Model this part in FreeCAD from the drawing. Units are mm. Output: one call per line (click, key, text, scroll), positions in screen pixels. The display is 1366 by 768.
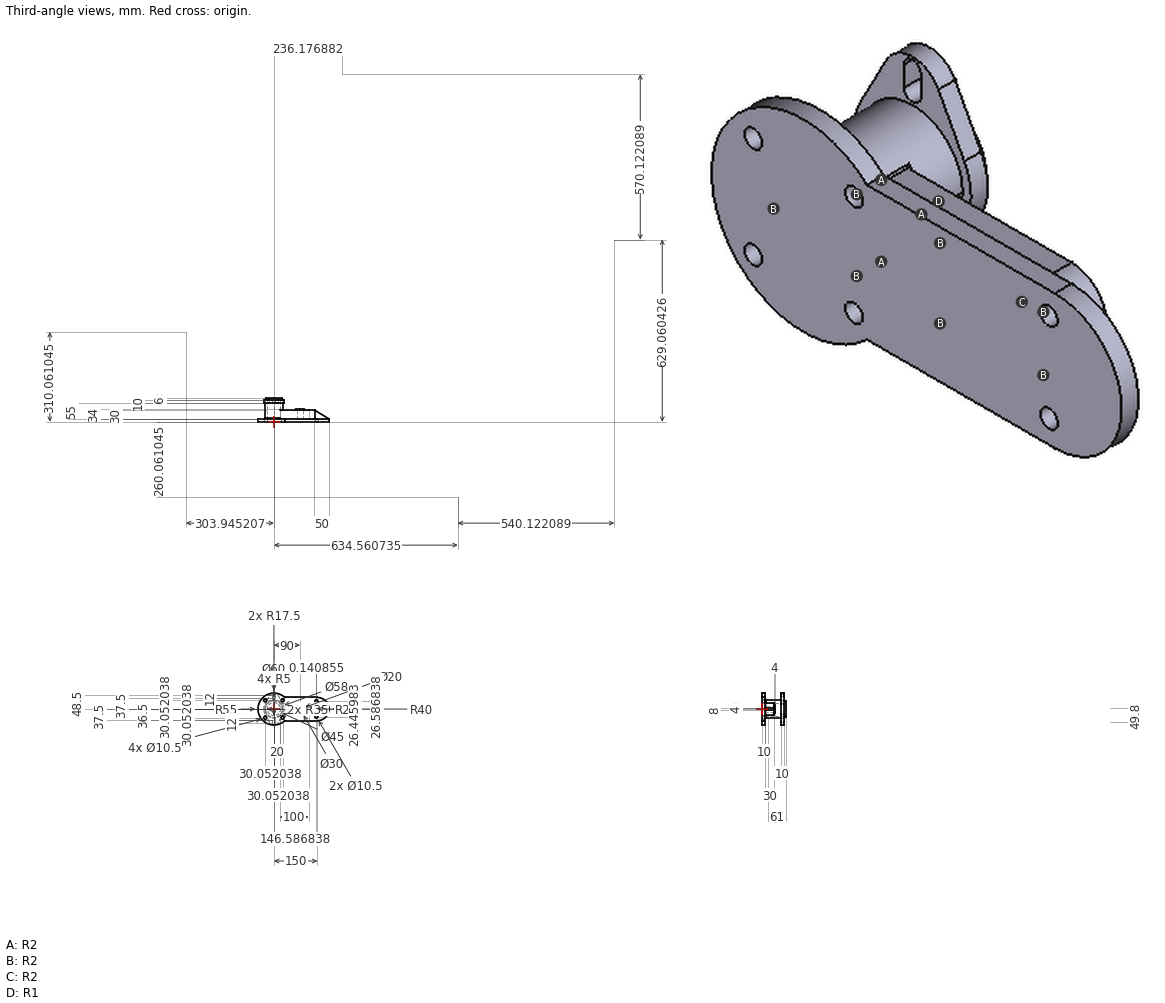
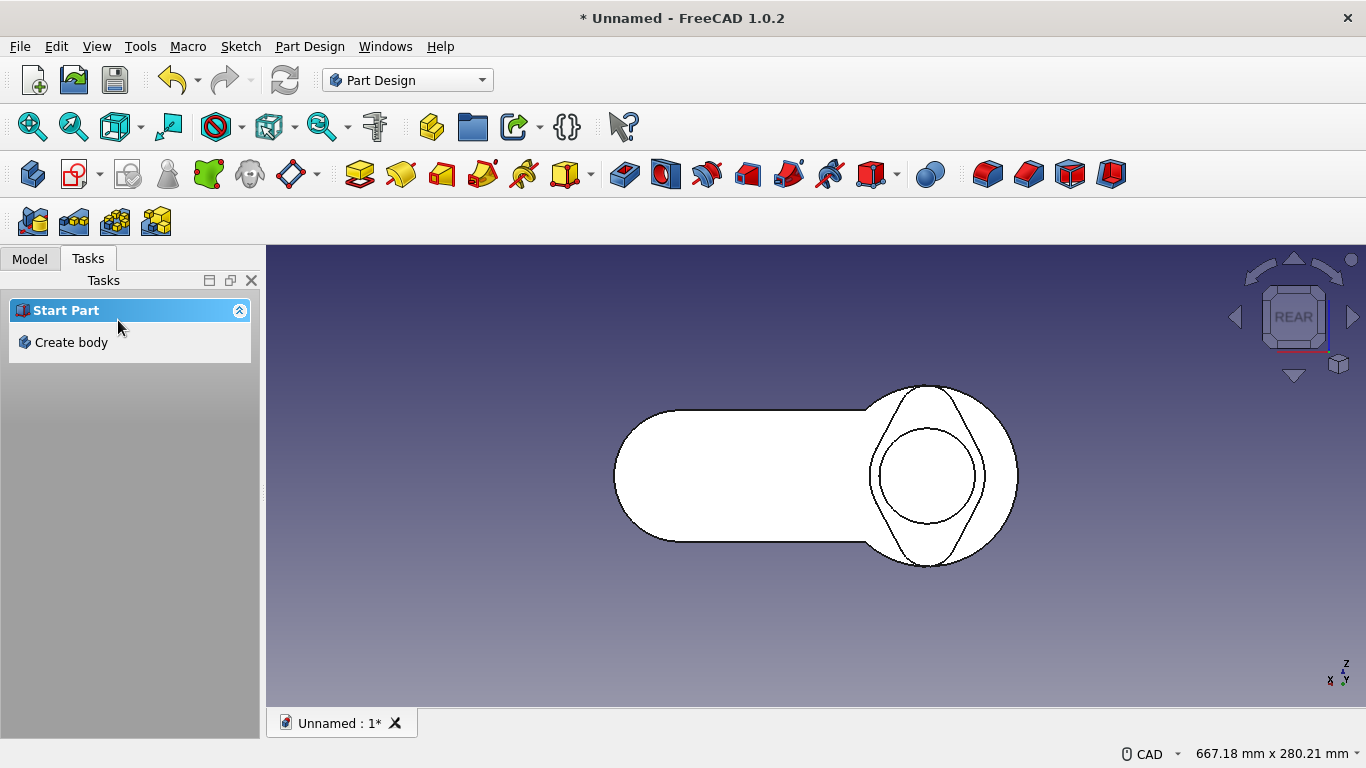
click(927, 475)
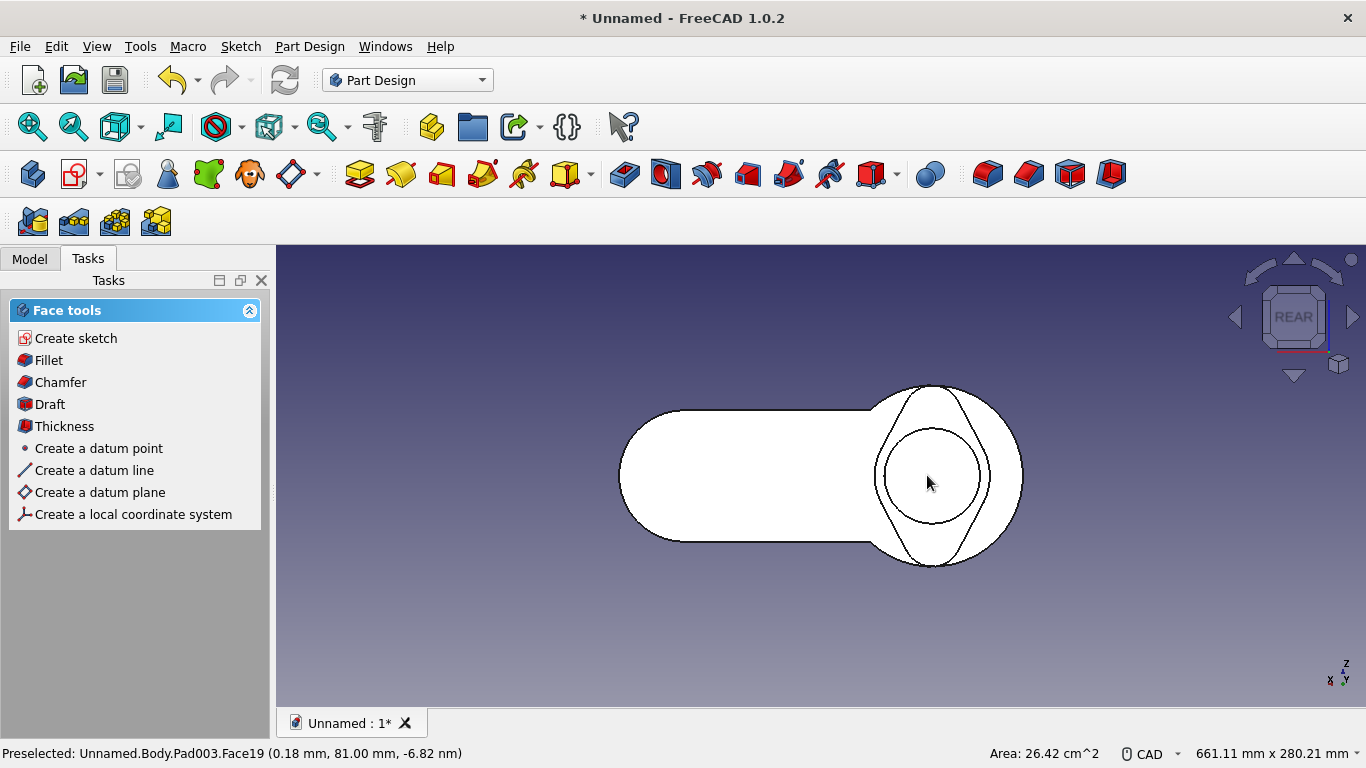
click(74, 174)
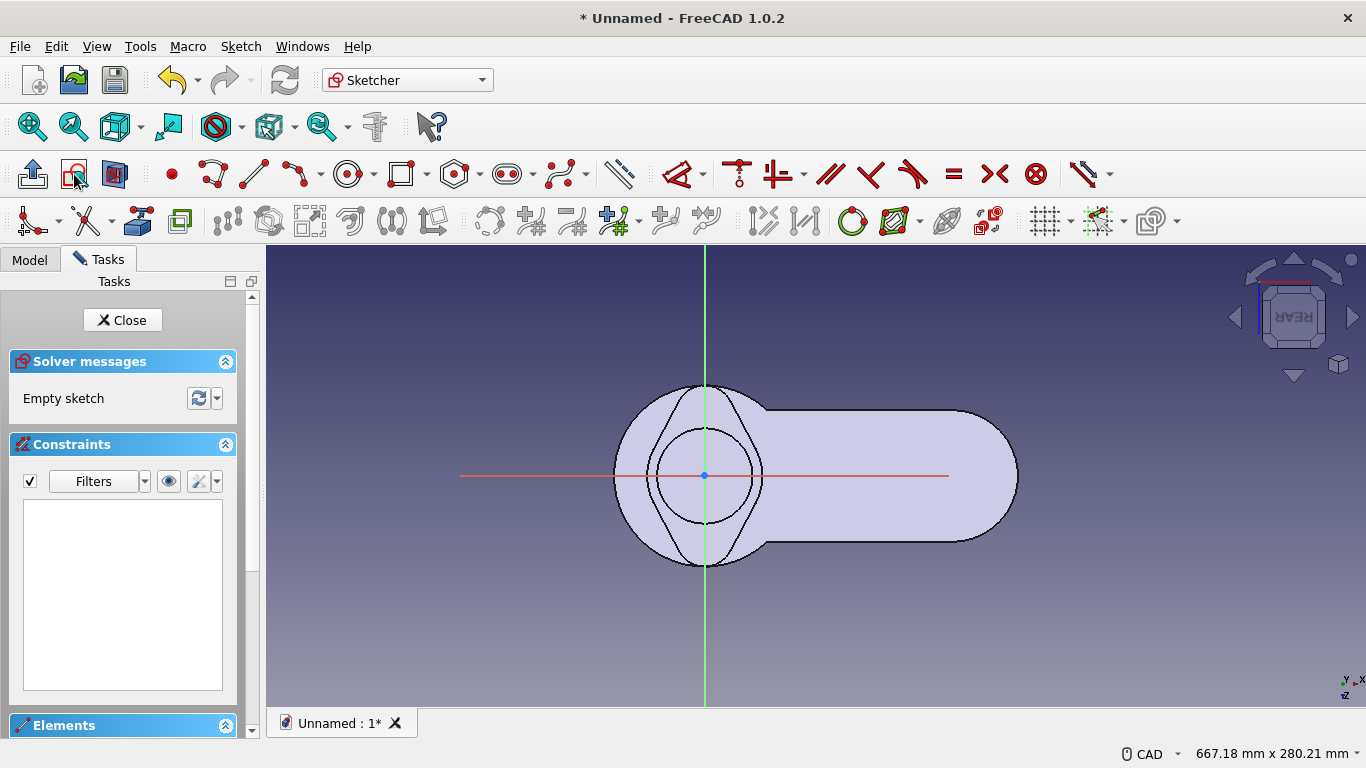
scroll(691, 476, up, 7)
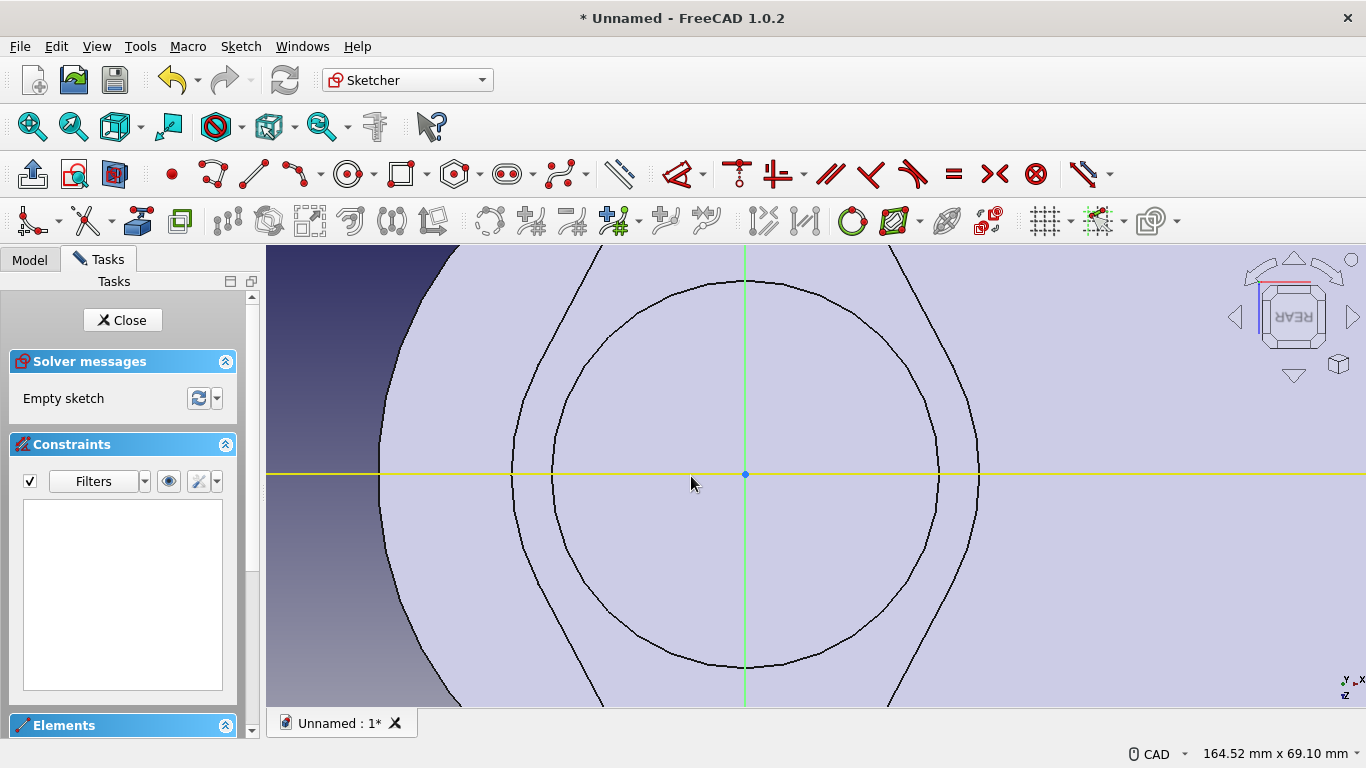
key(g)
key(c)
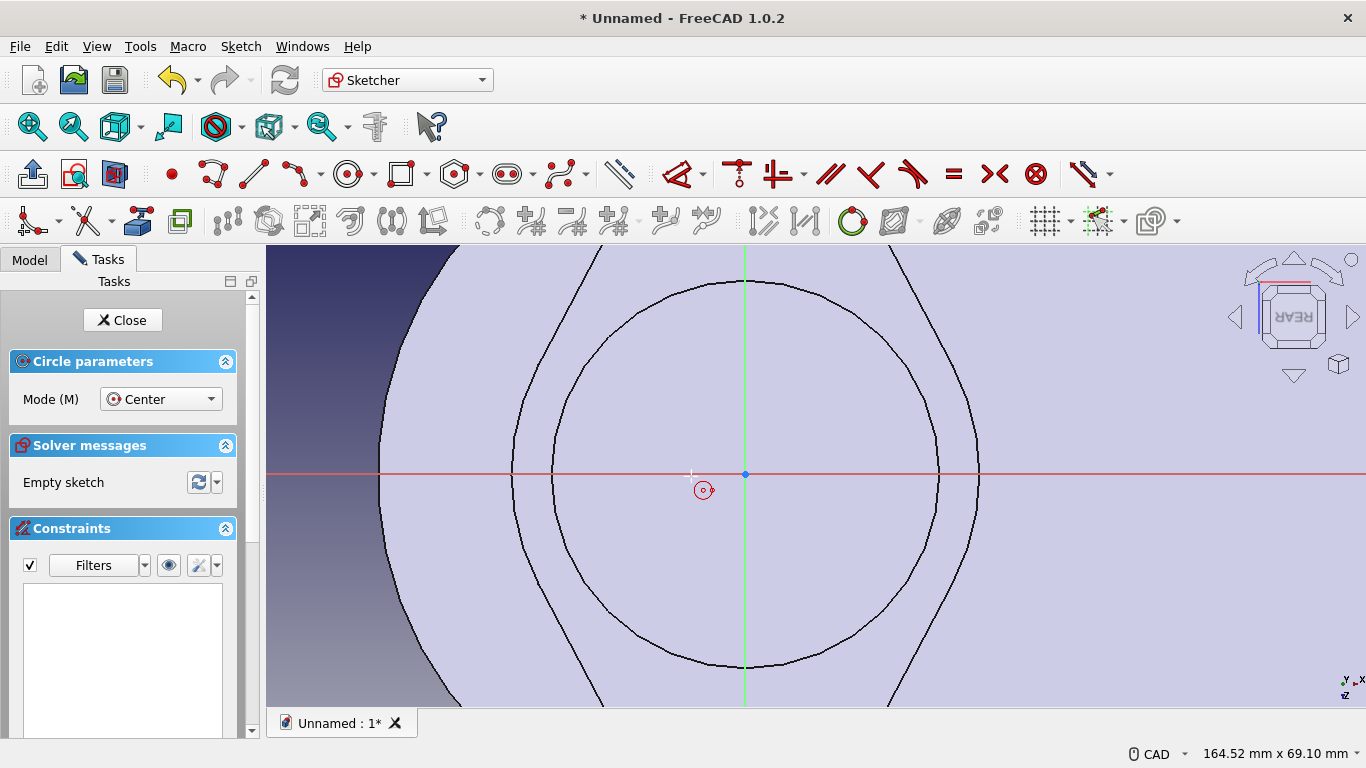
click(745, 474)
click(852, 368)
key(Escape)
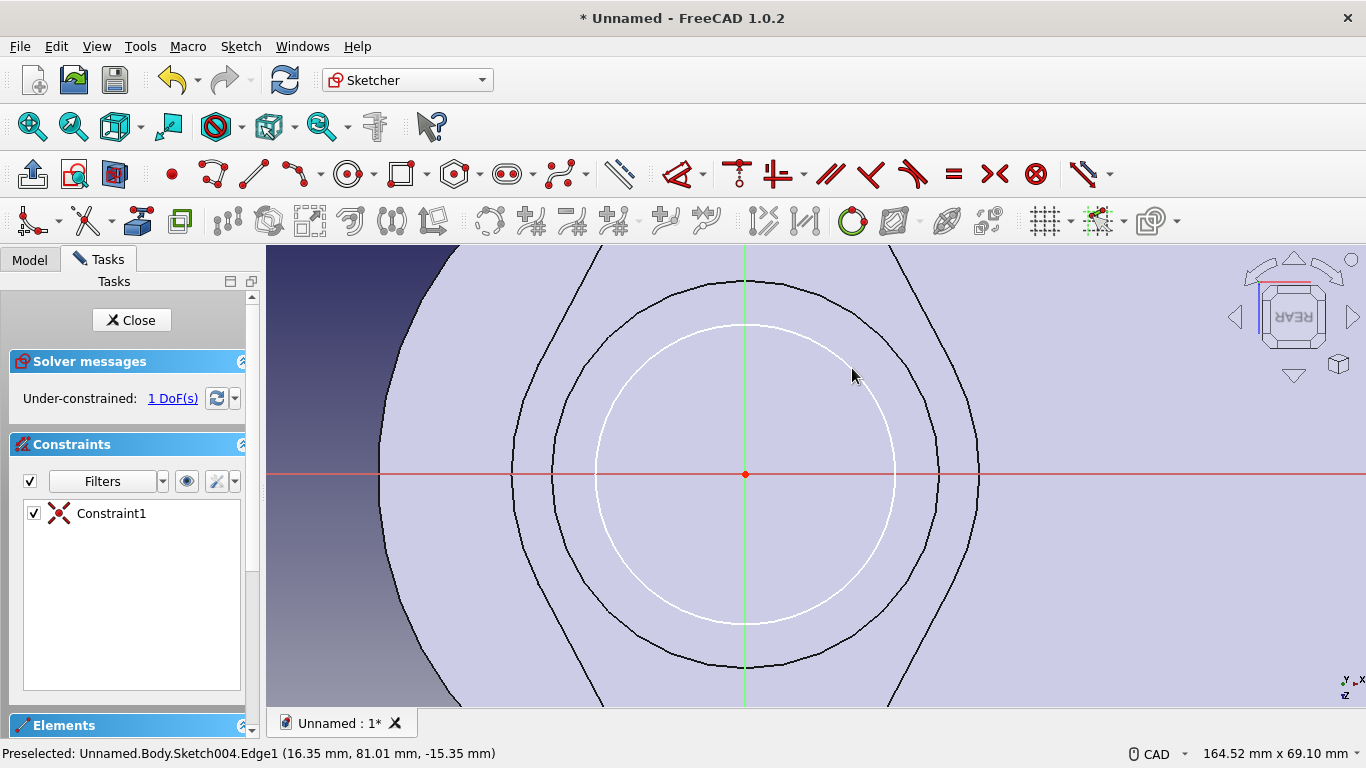
click(676, 174)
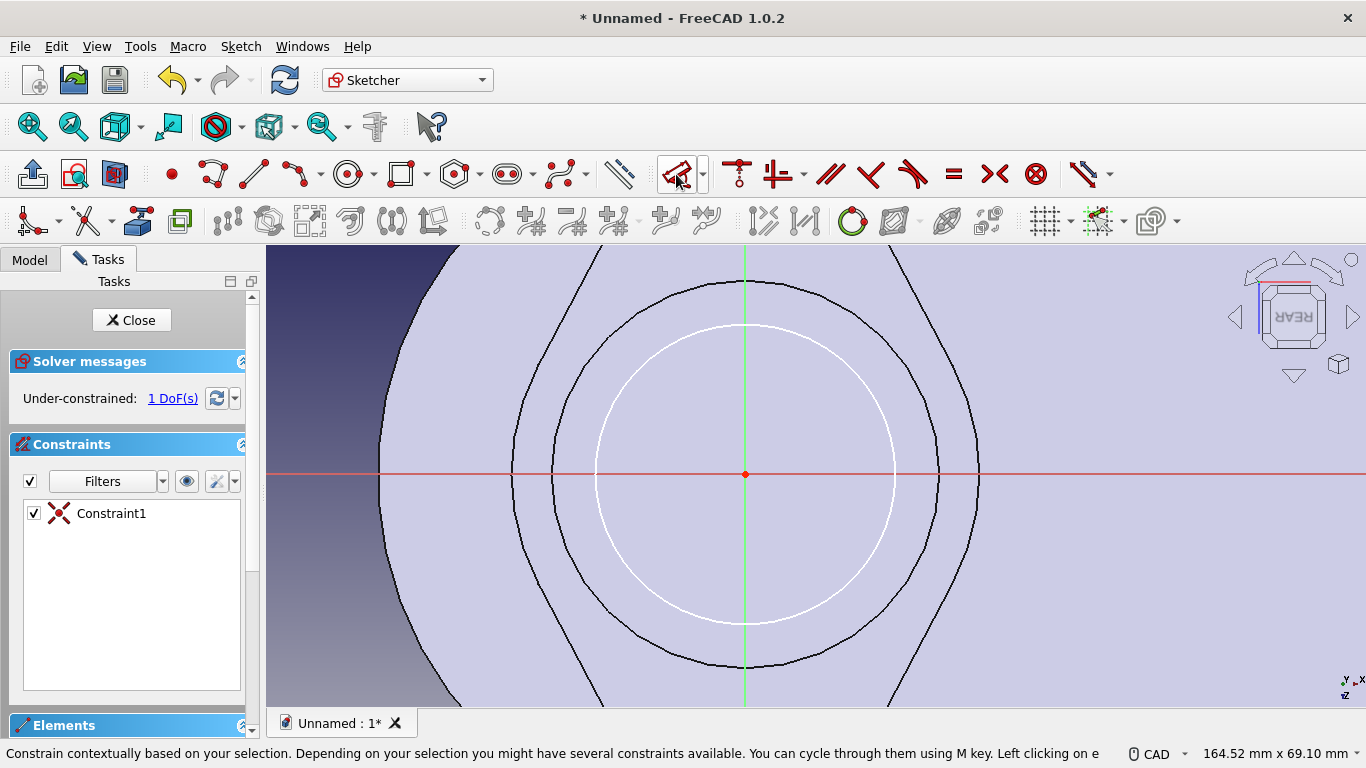
click(851, 368)
click(874, 345)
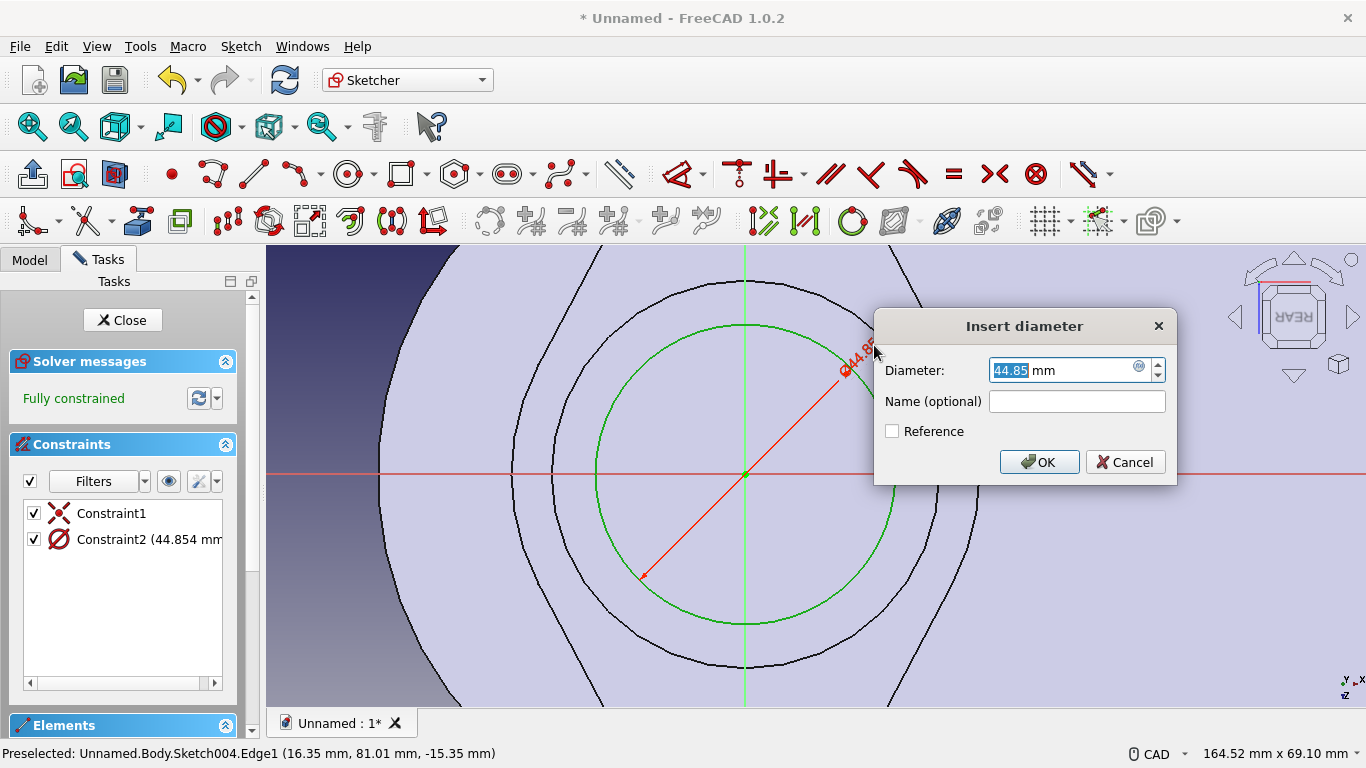
text(45)
key(Return)
key(Escape)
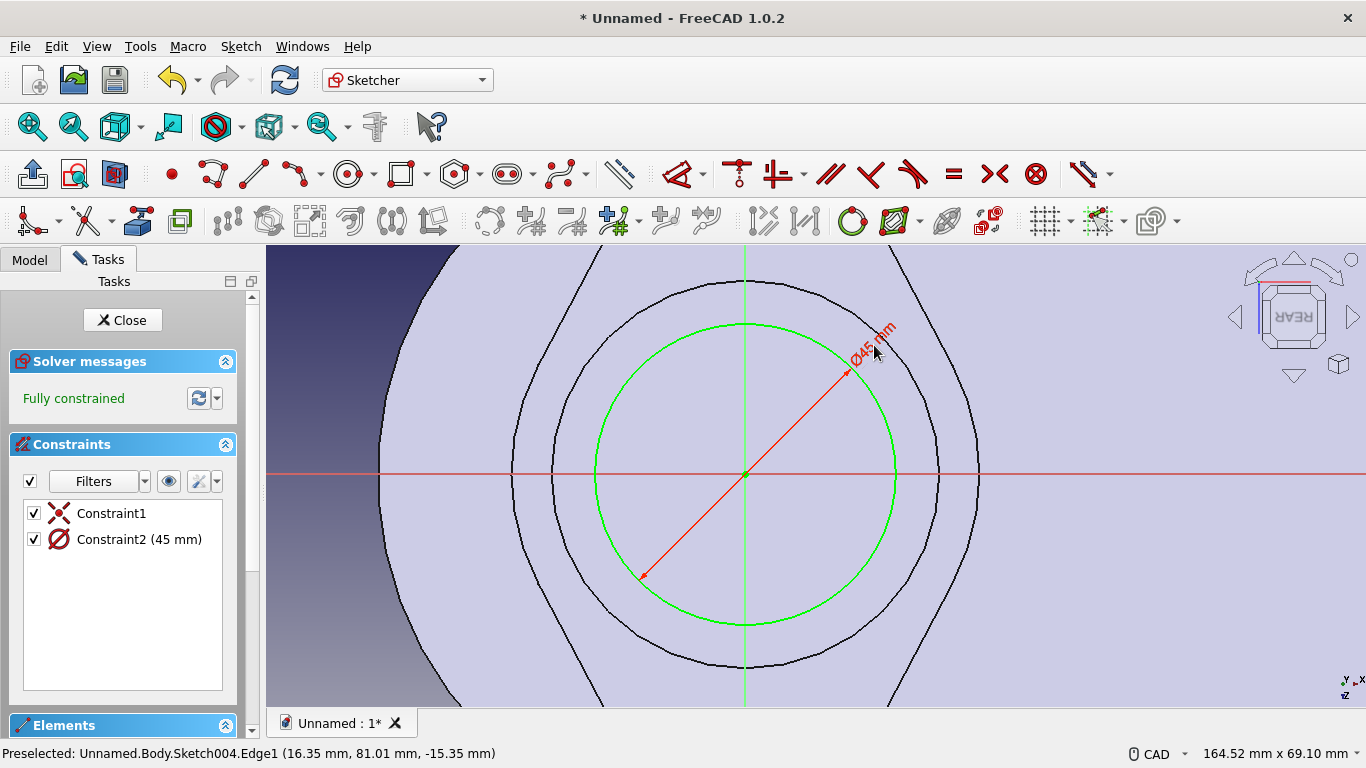
click(123, 320)